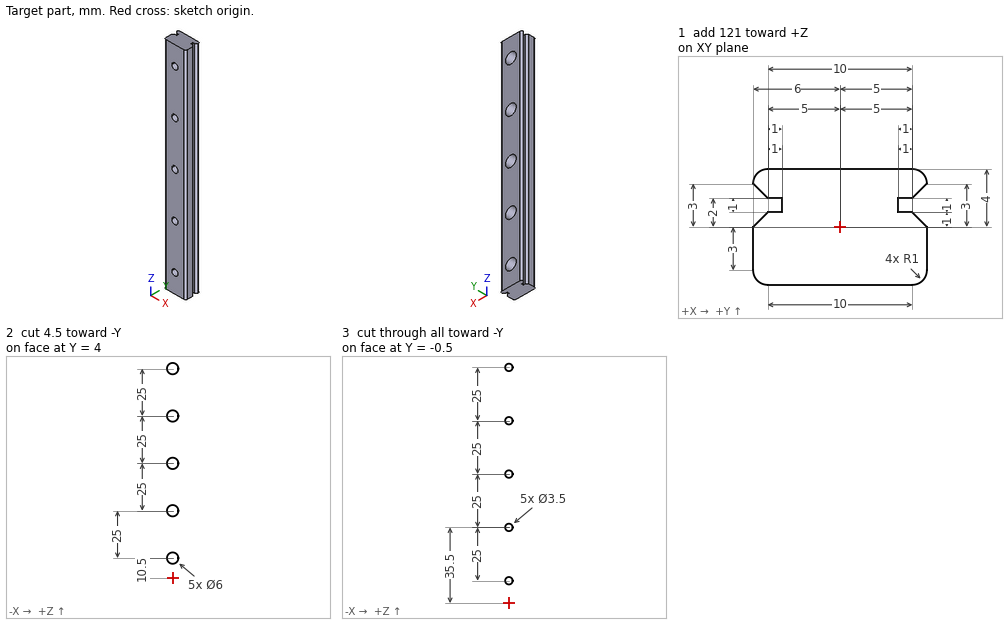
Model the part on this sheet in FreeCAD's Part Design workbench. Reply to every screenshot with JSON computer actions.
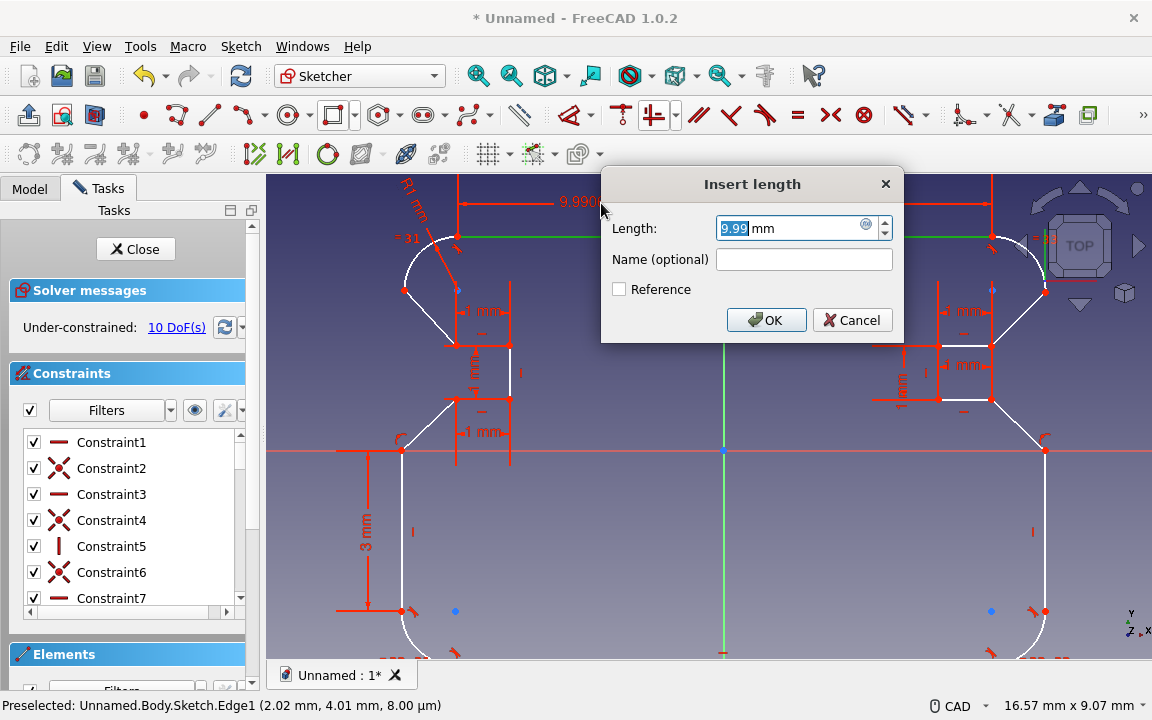
{"action": "type", "text": "10"}
{"action": "key", "text": "Return"}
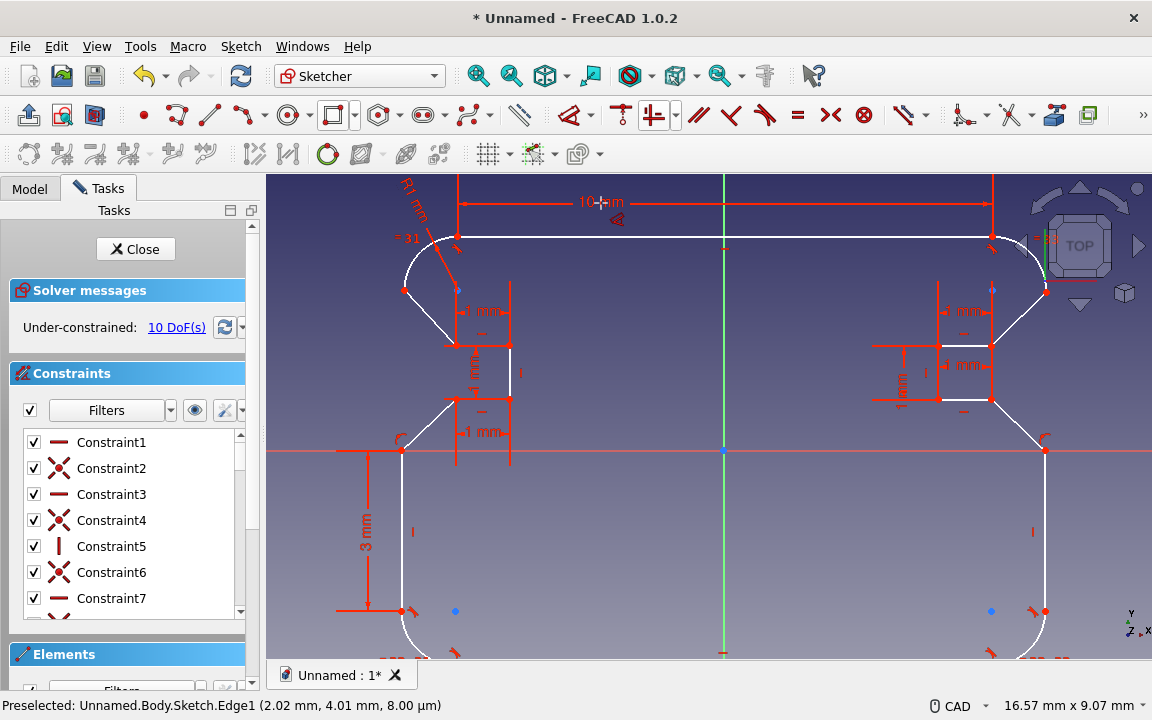
{"action": "scroll", "coordinate": [471, 346], "scroll_direction": "down", "scroll_amount": 2}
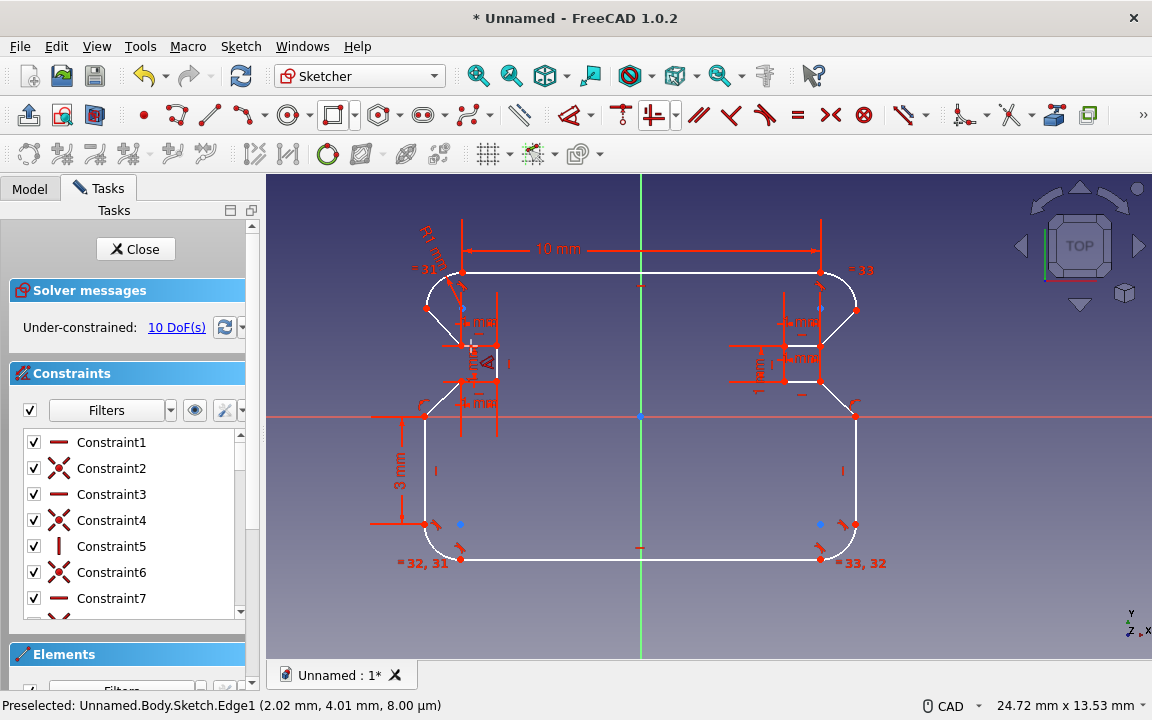
{"action": "left_click", "coordinate": [568, 560]}
{"action": "left_click", "coordinate": [558, 594]}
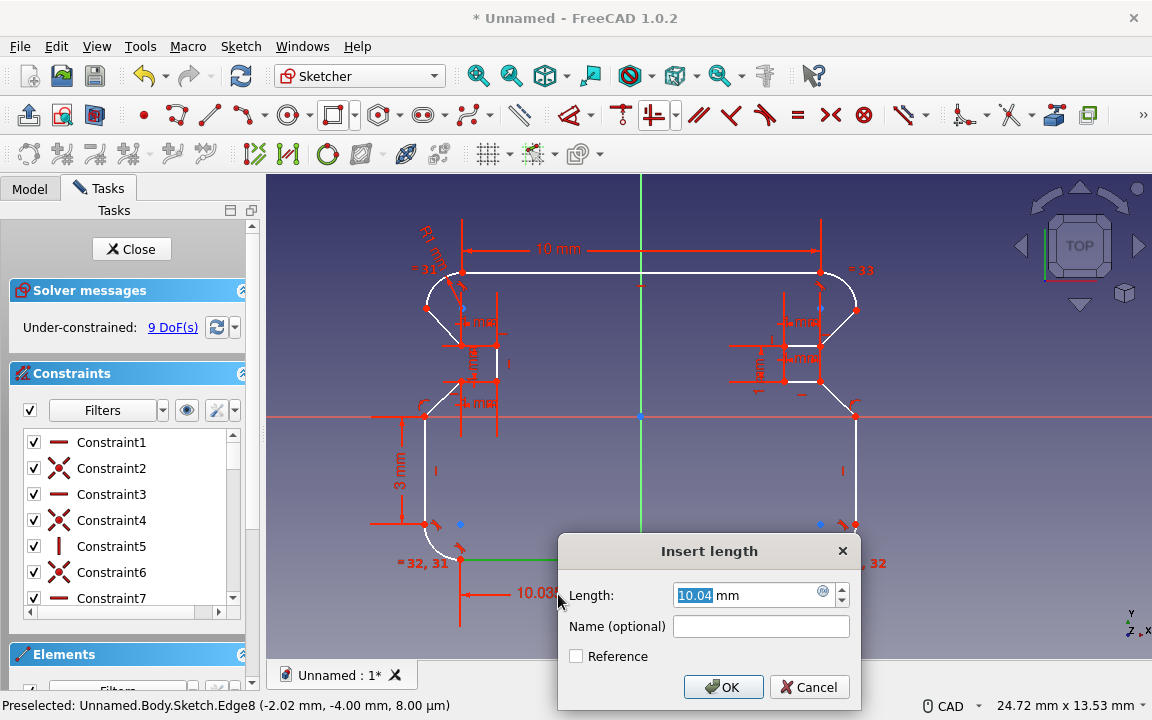
{"action": "type", "text": "10"}
{"action": "key", "text": "Return"}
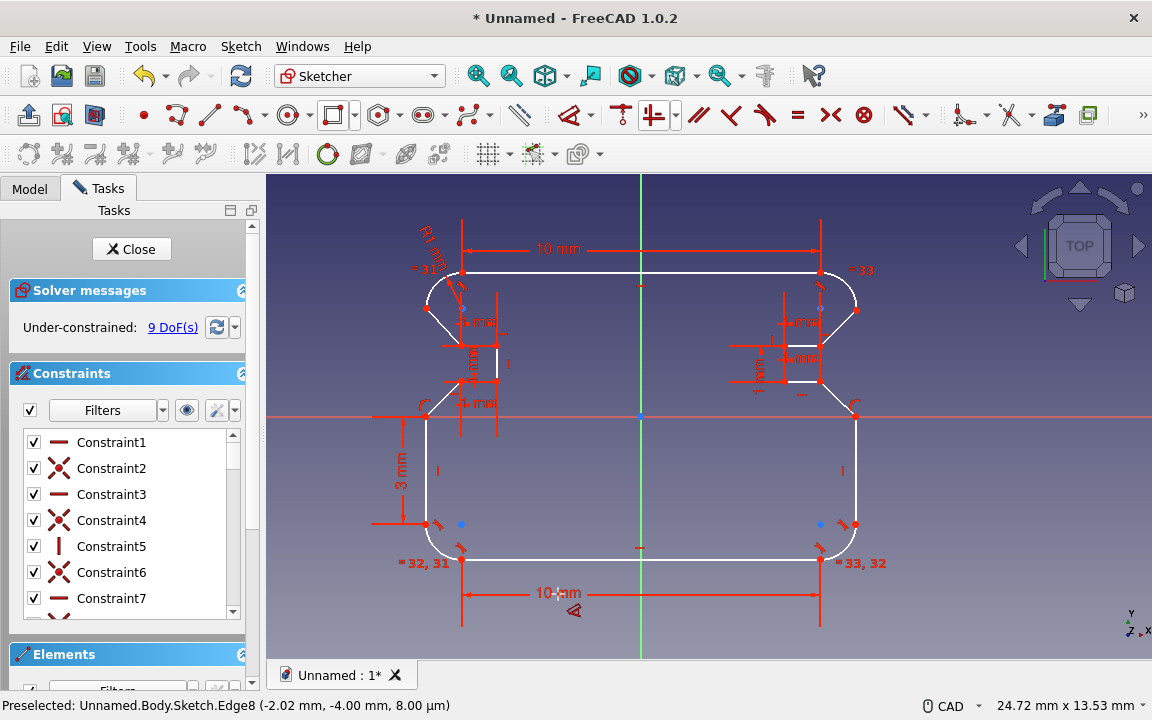
{"action": "left_click", "coordinate": [821, 273]}
{"action": "left_click", "coordinate": [731, 239]}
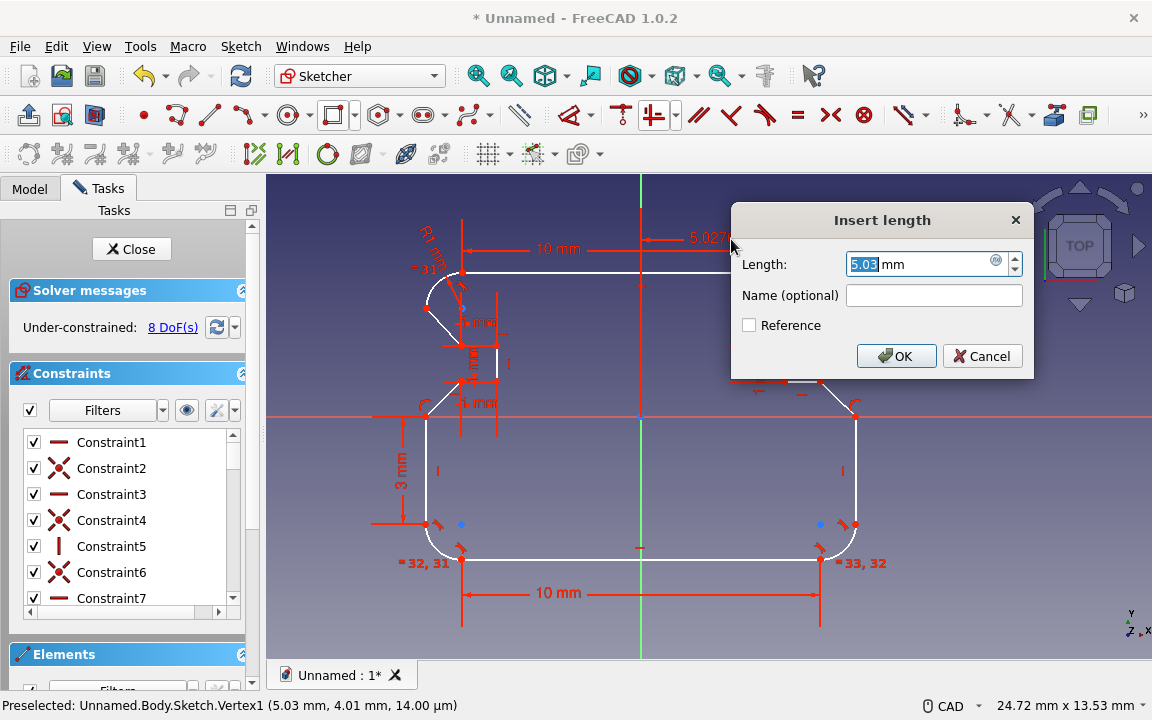
{"action": "type", "text": "5"}
{"action": "key", "text": "Return"}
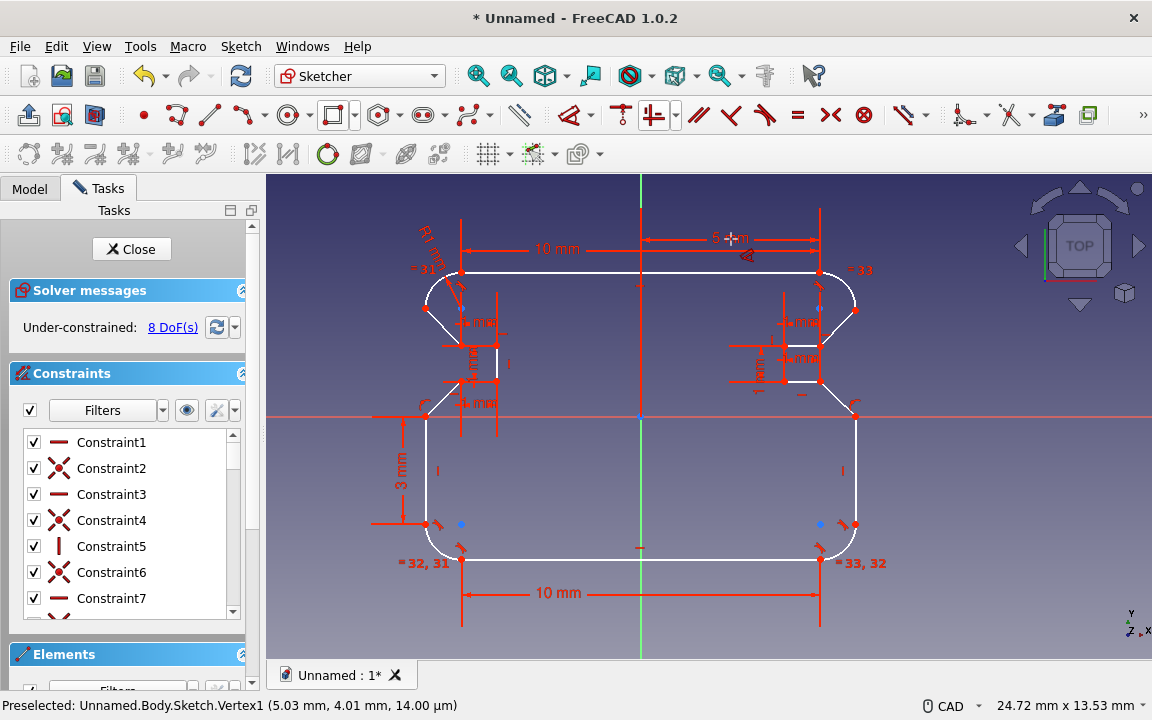
{"action": "left_click", "coordinate": [820, 273]}
{"action": "left_click", "coordinate": [854, 395]}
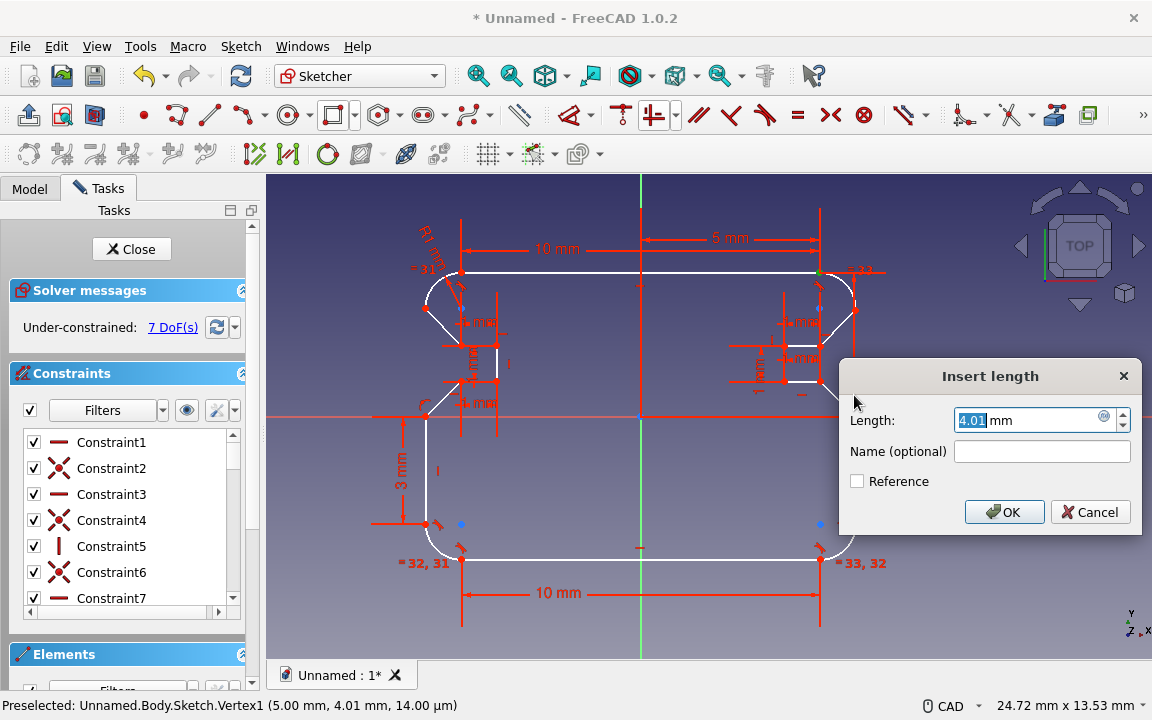
{"action": "type", "text": "4"}
{"action": "key", "text": "Return"}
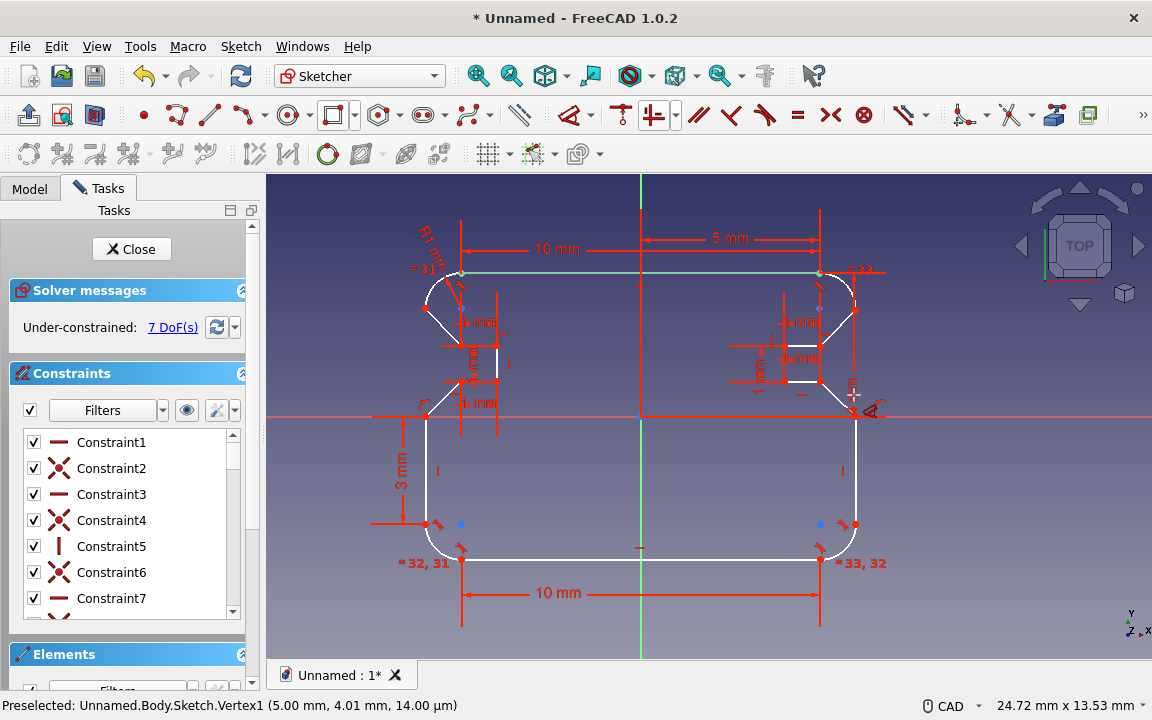
{"action": "left_click", "coordinate": [426, 309]}
{"action": "left_click", "coordinate": [392, 363]}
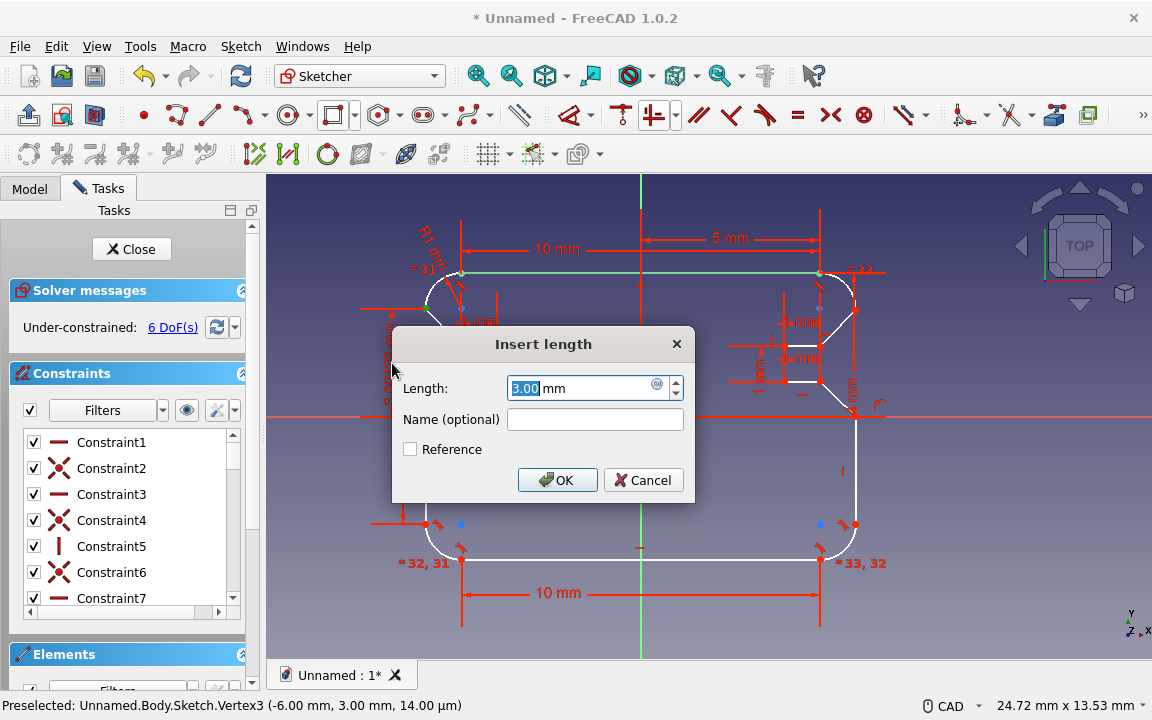
{"action": "type", "text": "3"}
{"action": "key", "text": "Return"}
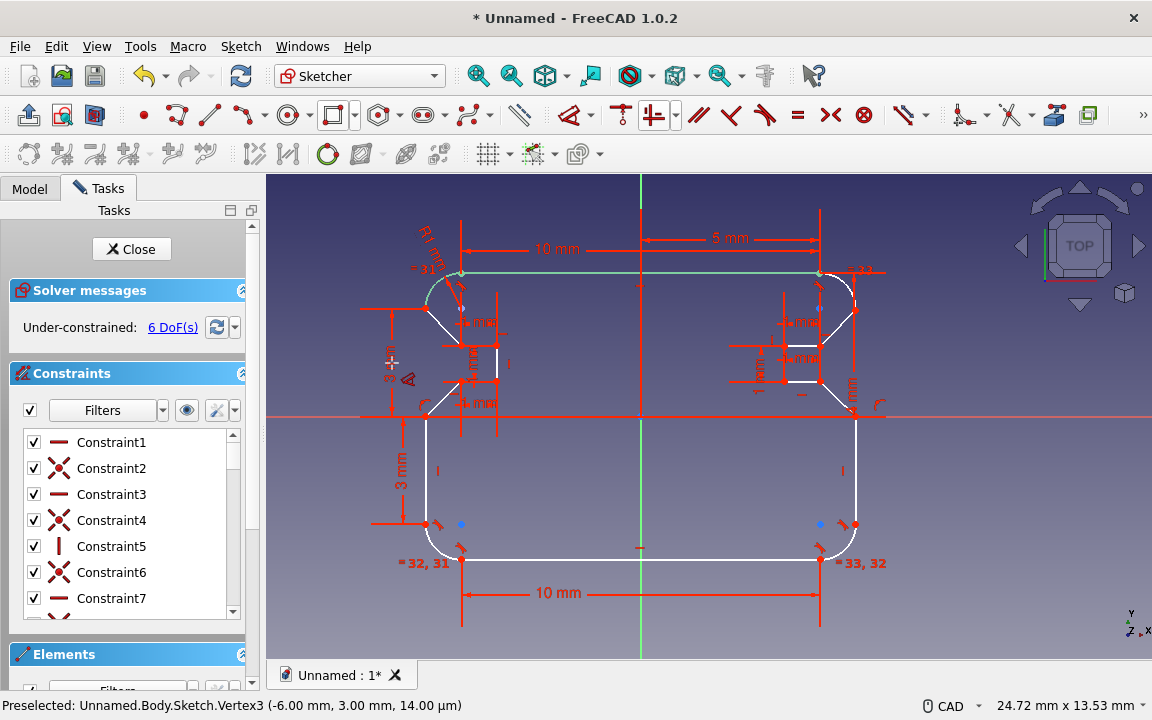
{"action": "left_click", "coordinate": [461, 346]}
{"action": "left_click", "coordinate": [551, 312]}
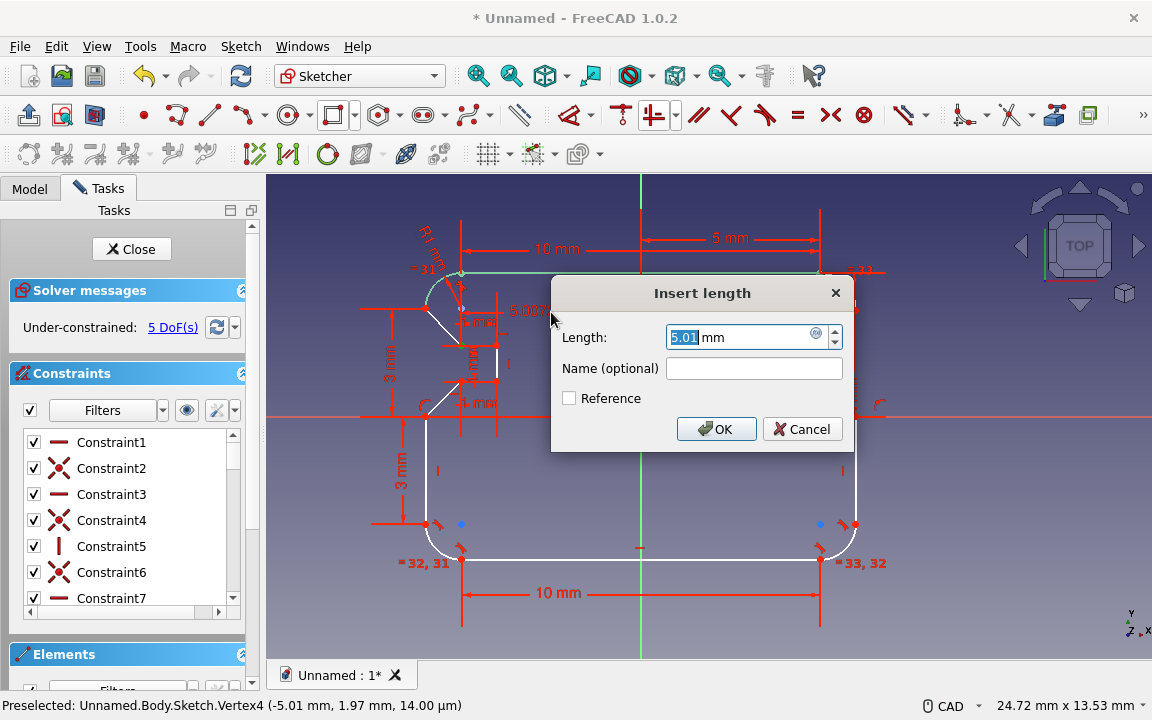
{"action": "type", "text": "5"}
{"action": "key", "text": "Return"}